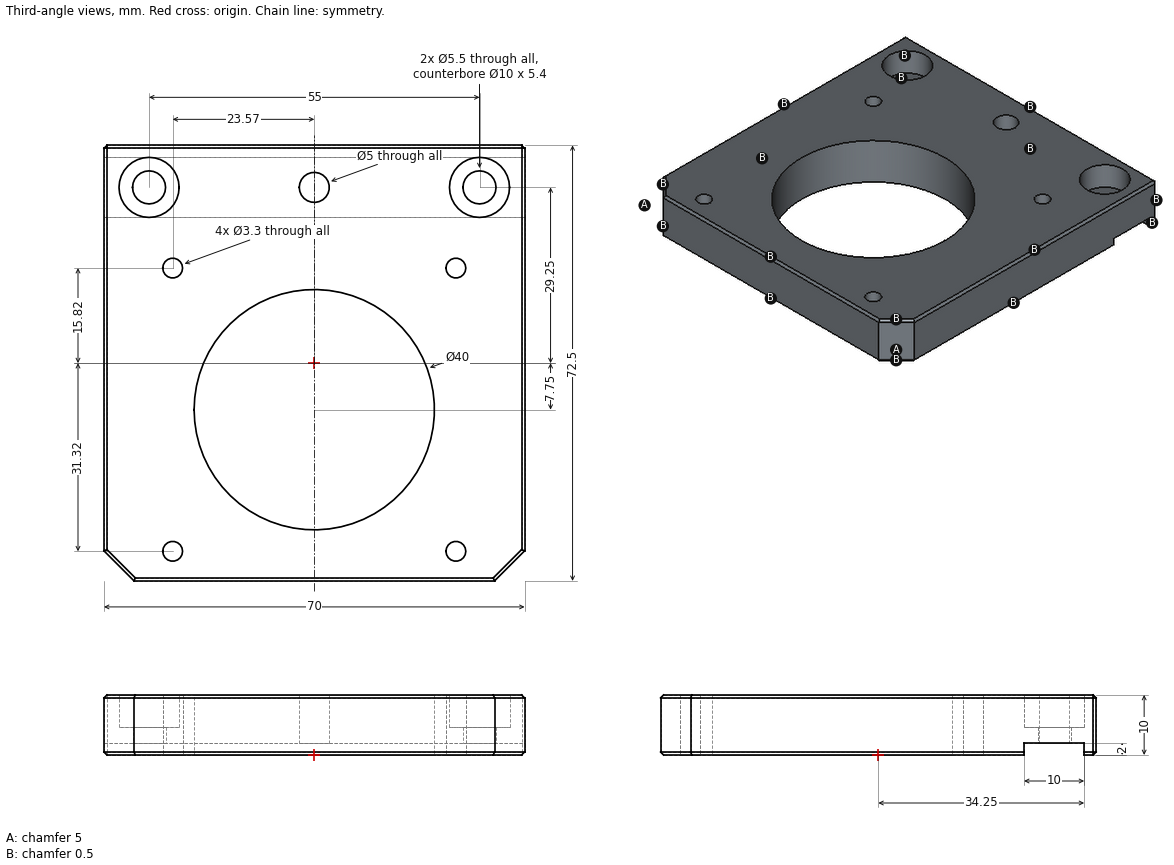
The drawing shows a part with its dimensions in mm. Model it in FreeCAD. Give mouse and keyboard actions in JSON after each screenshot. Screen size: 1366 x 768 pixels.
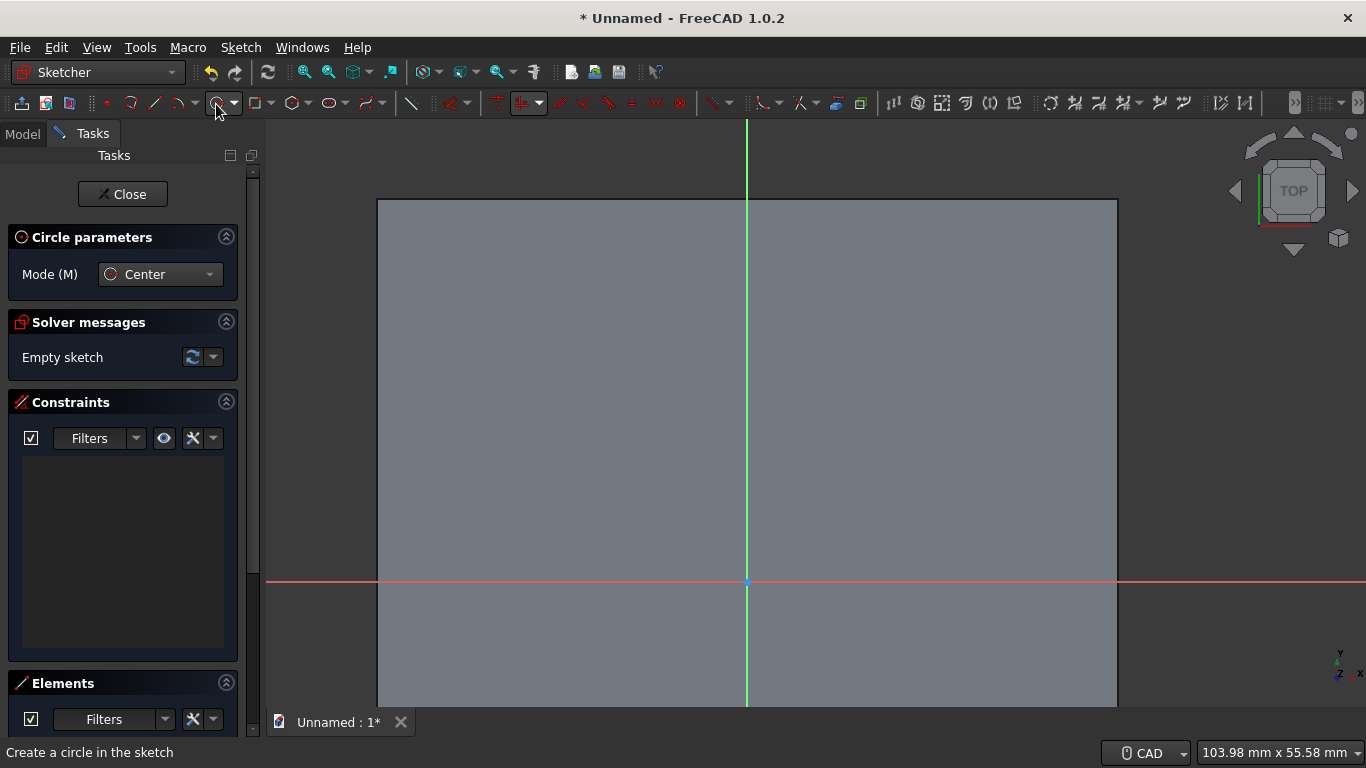
{"action": "left_click", "coordinate": [1038, 273]}
{"action": "mouse_move", "coordinate": [1059, 252]}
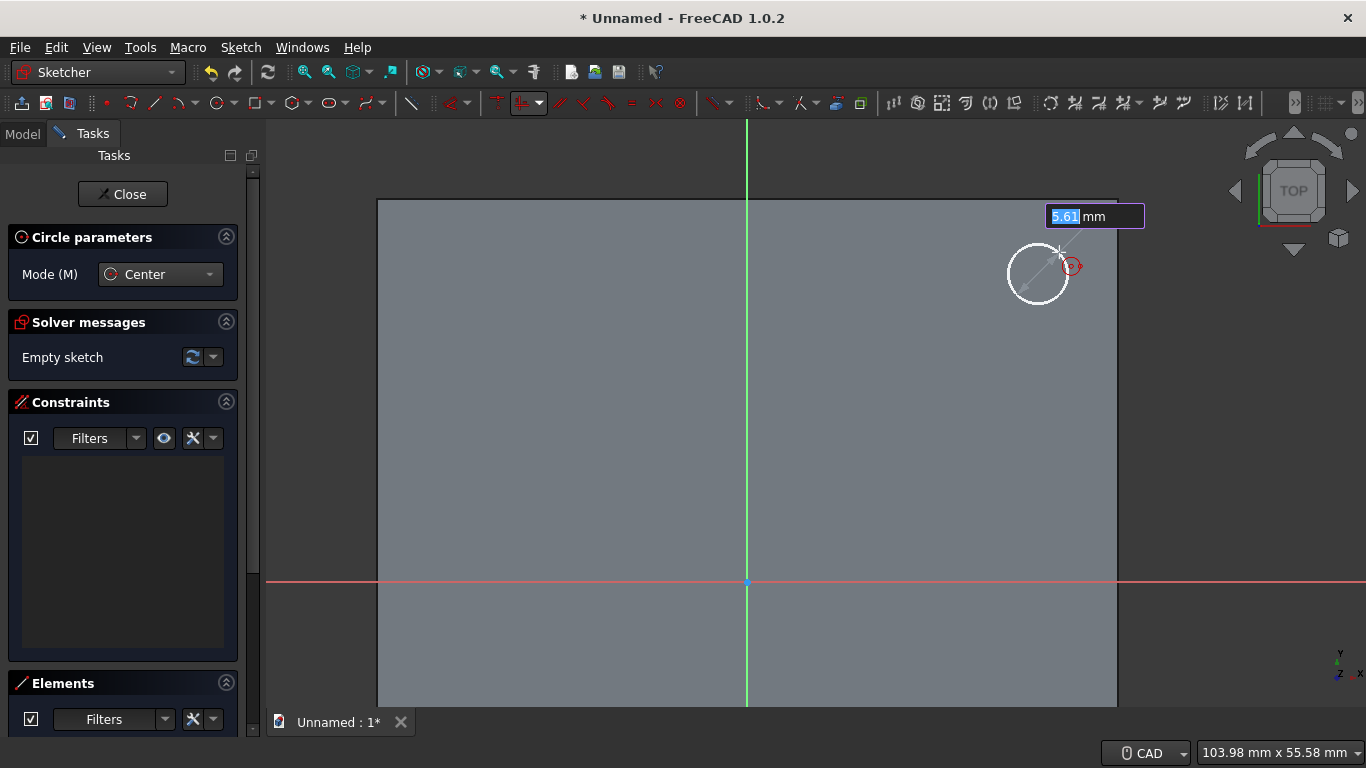
{"action": "type", "text": "5.5"}
{"action": "key", "text": "Return"}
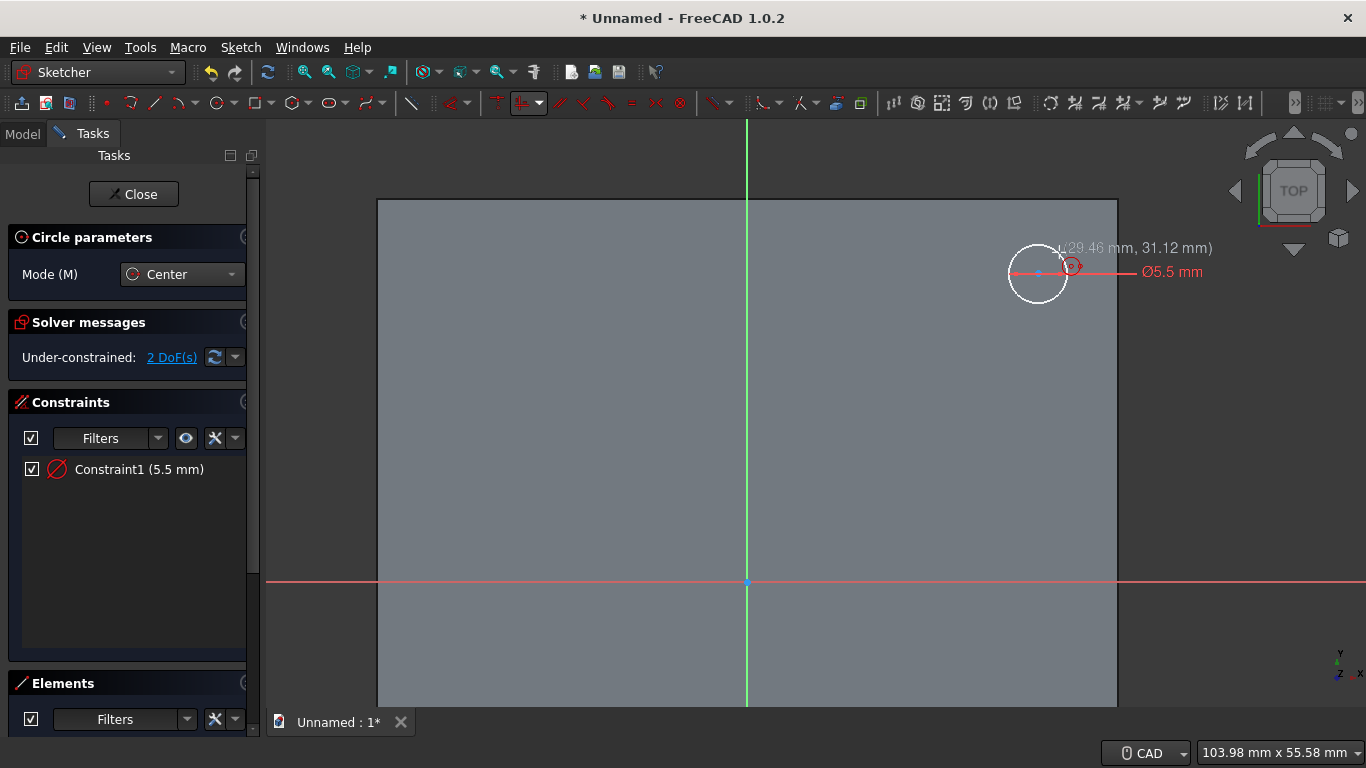
{"action": "left_click", "coordinate": [456, 273]}
{"action": "mouse_move", "coordinate": [477, 252]}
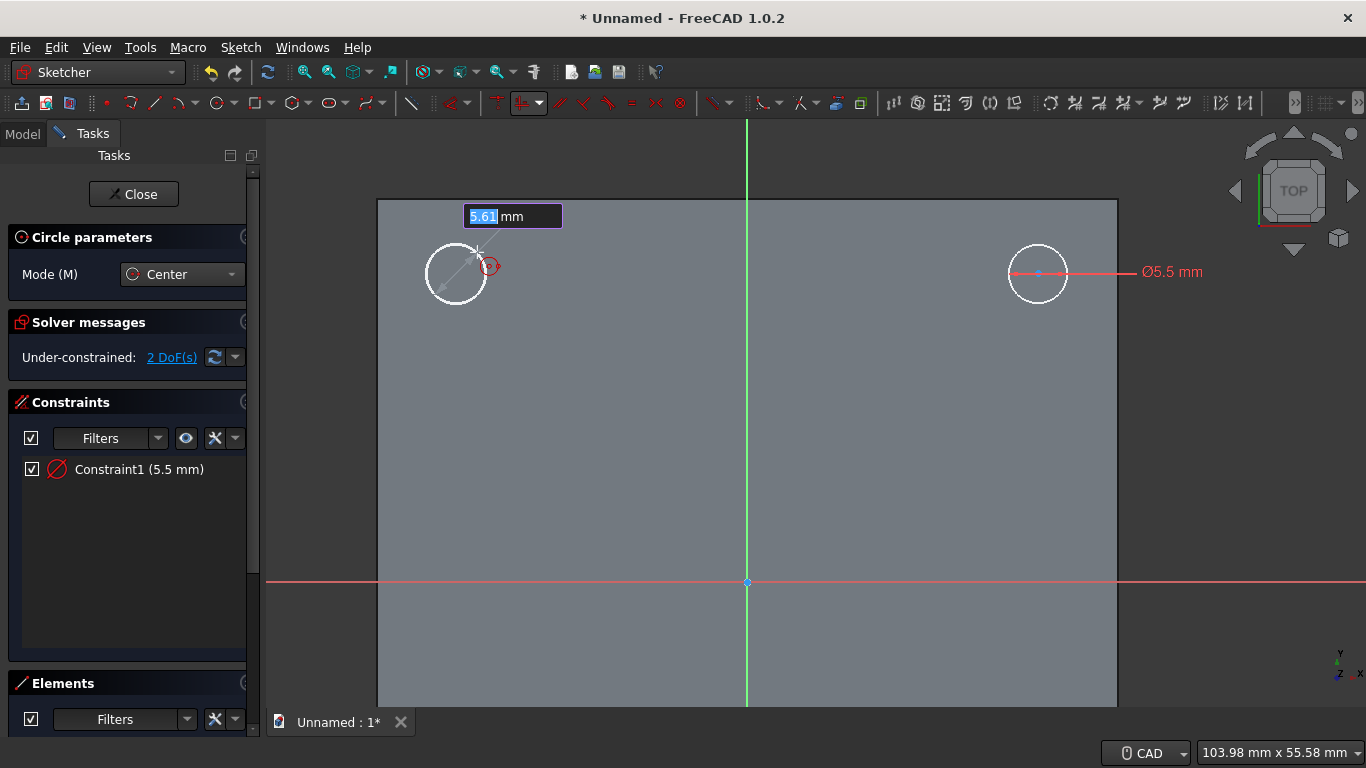
{"action": "type", "text": "5.5"}
{"action": "key", "text": "Return"}
{"action": "key", "text": "Escape"}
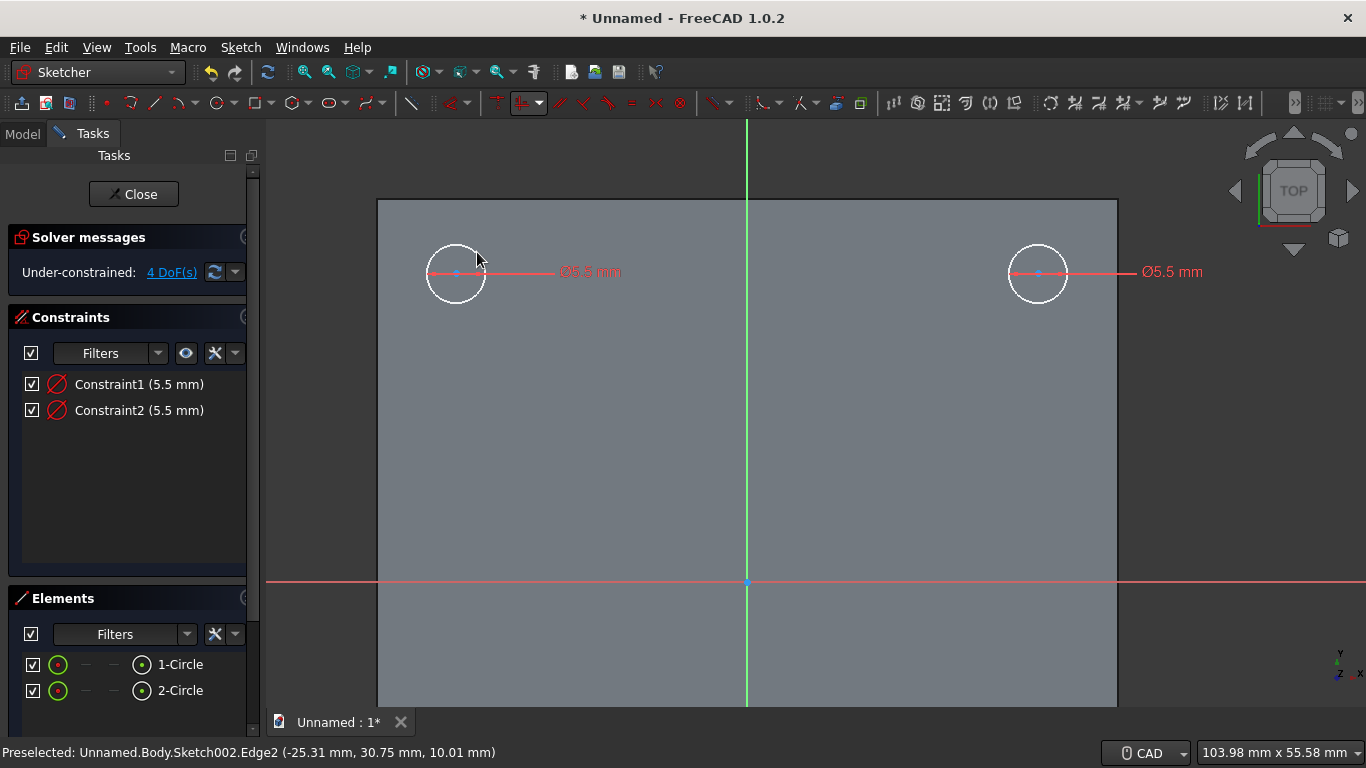
{"action": "left_click", "coordinate": [1038, 274]}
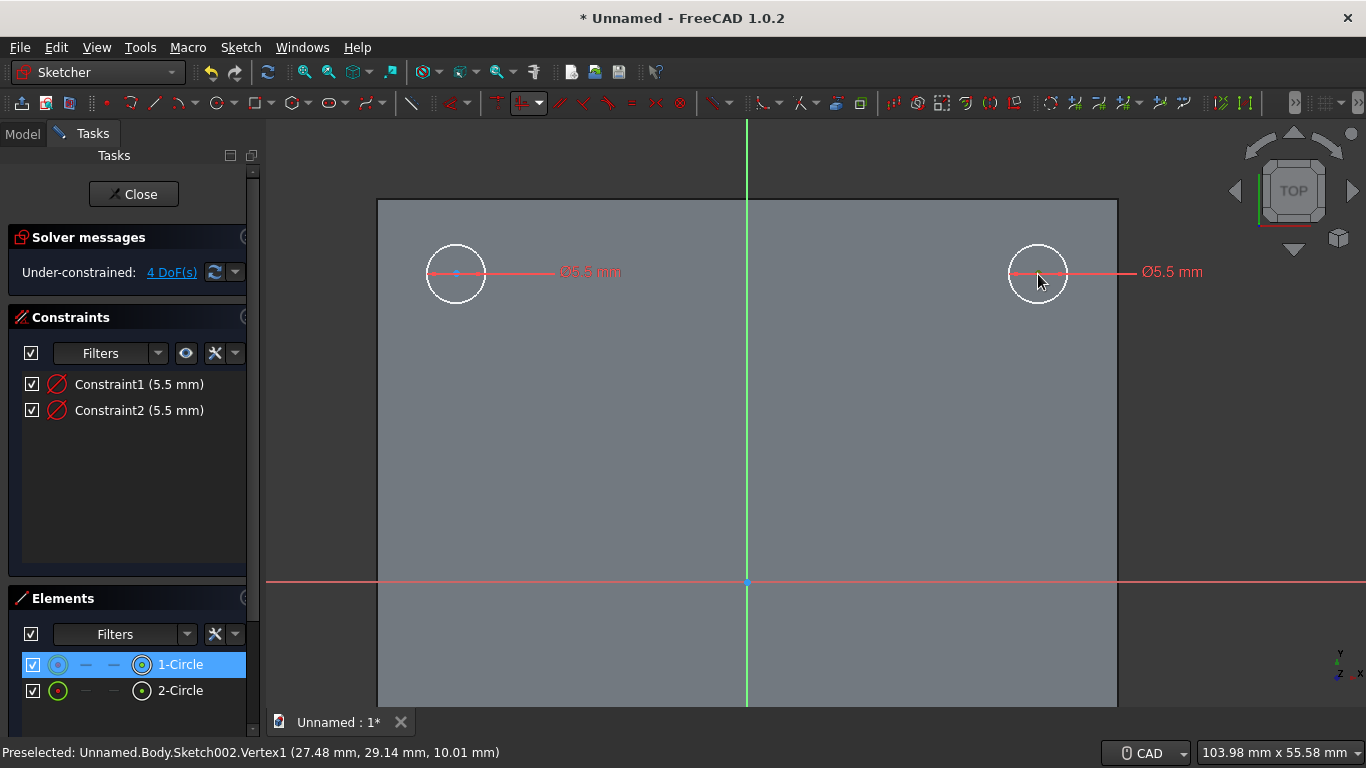
{"action": "left_click", "coordinate": [456, 274]}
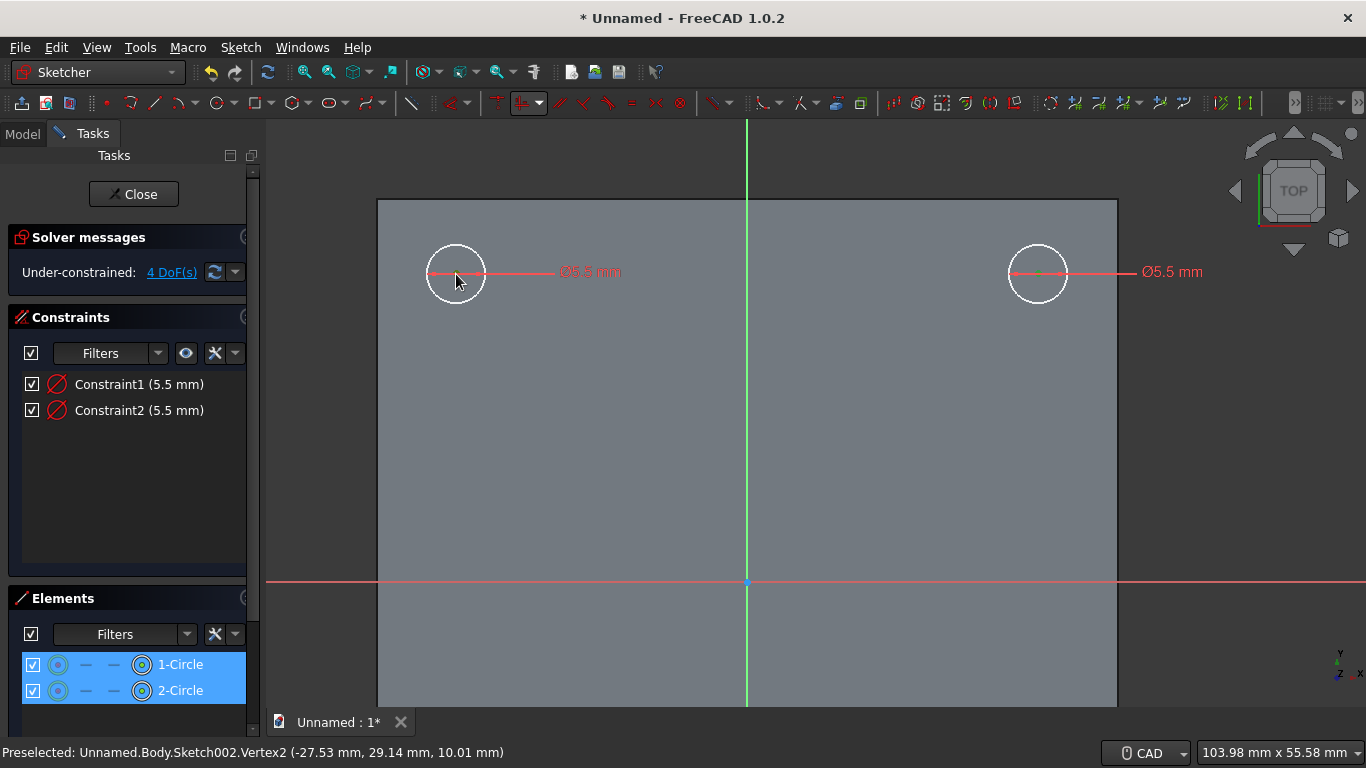
{"action": "left_click", "coordinate": [747, 641]}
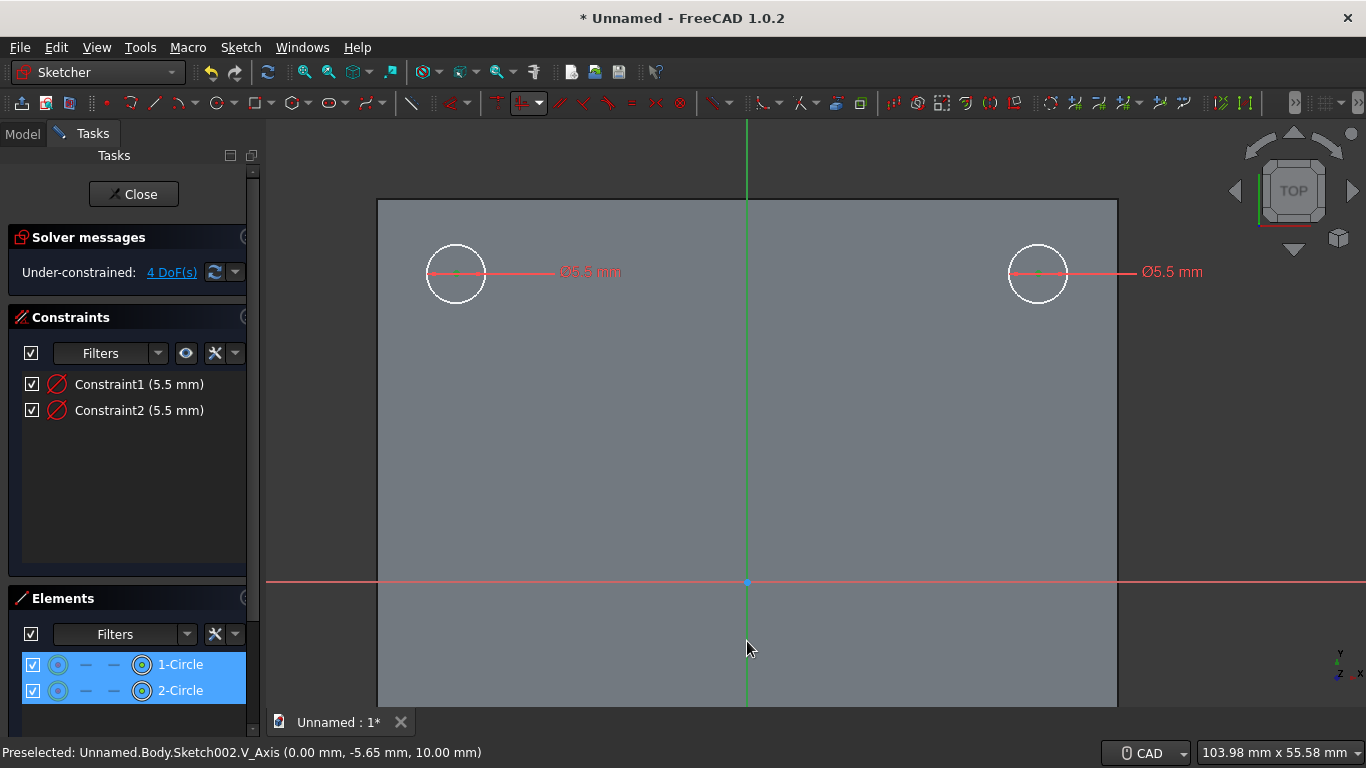
{"action": "left_click", "coordinate": [656, 104]}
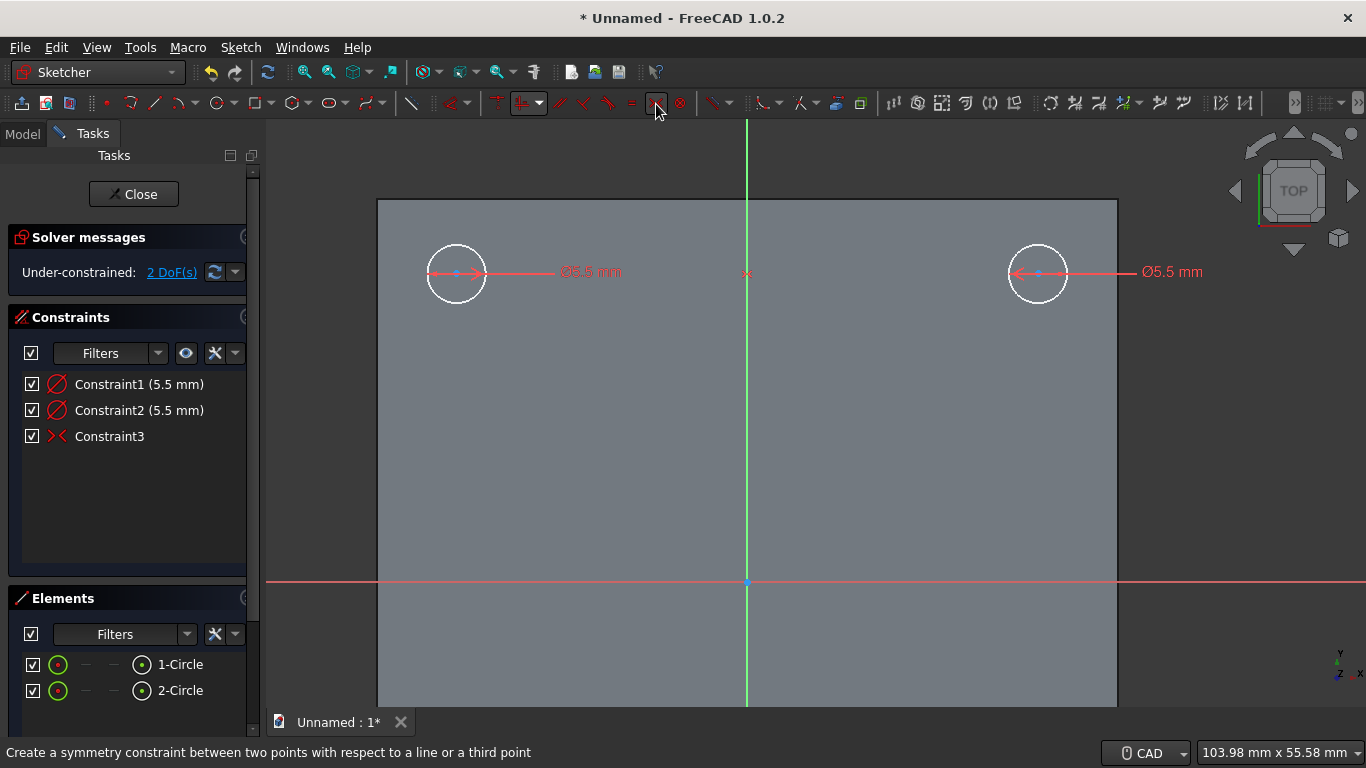
{"action": "left_click", "coordinate": [450, 104]}